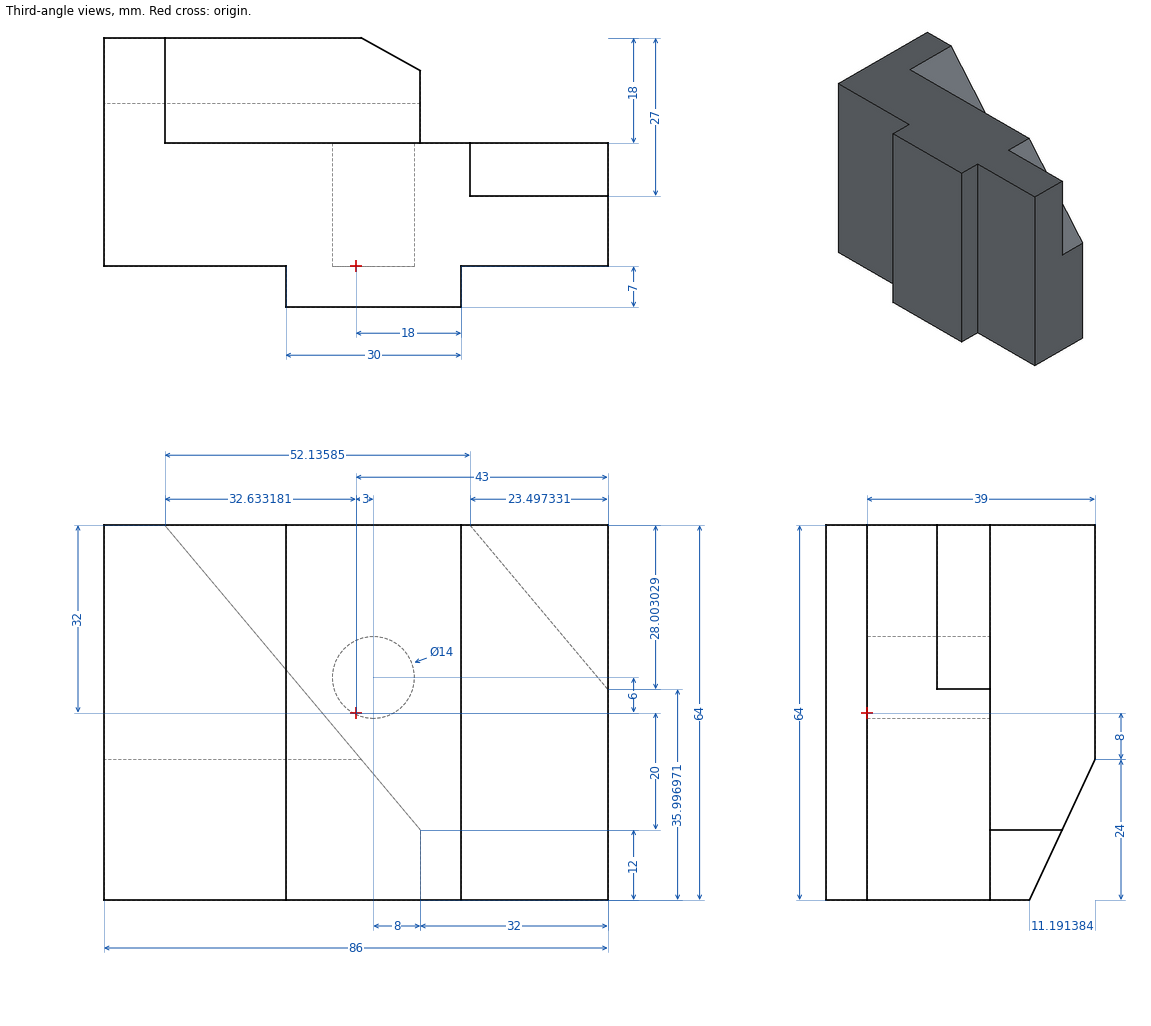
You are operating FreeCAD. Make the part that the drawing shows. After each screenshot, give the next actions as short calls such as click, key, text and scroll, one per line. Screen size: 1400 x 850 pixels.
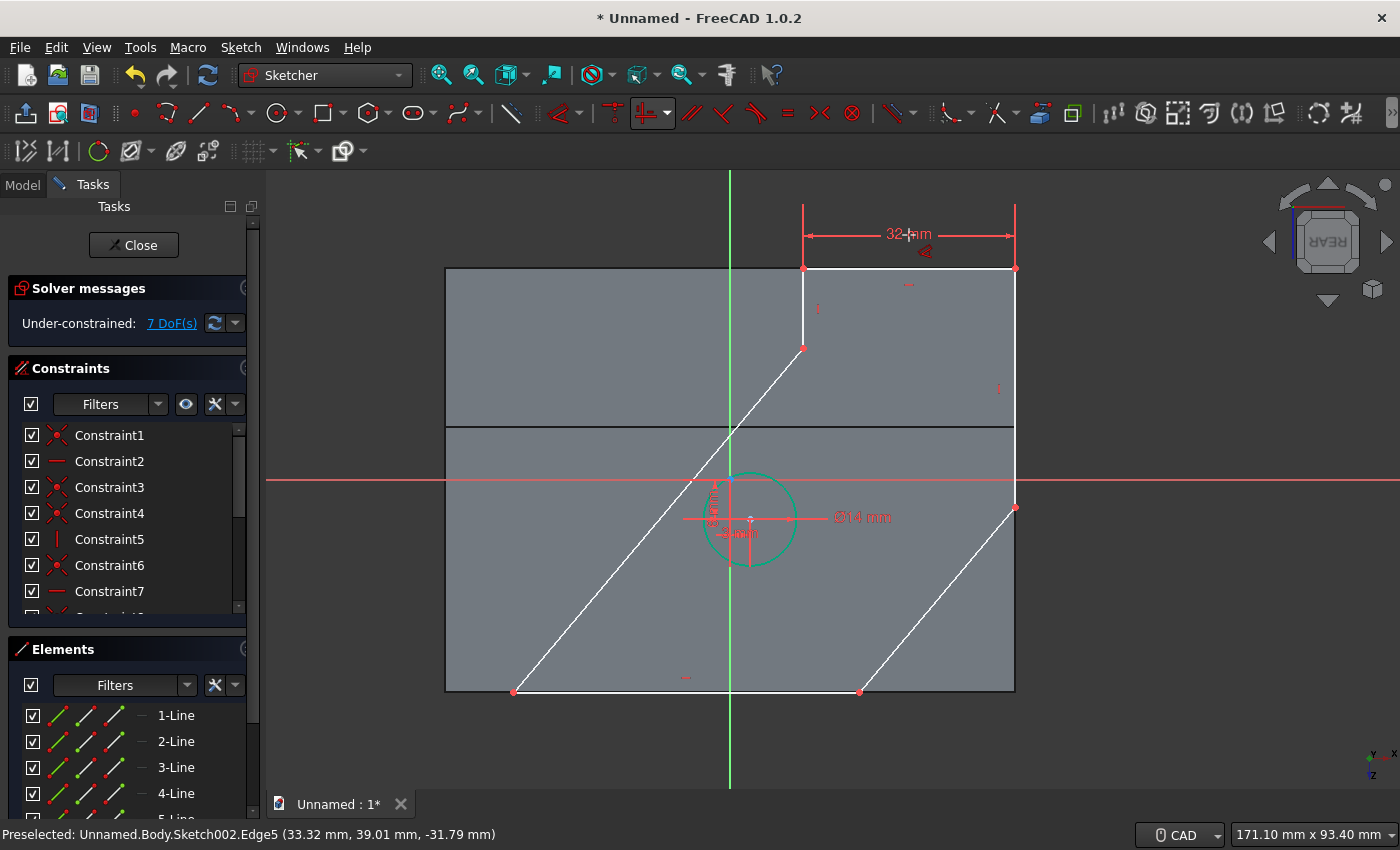
click(803, 293)
click(837, 309)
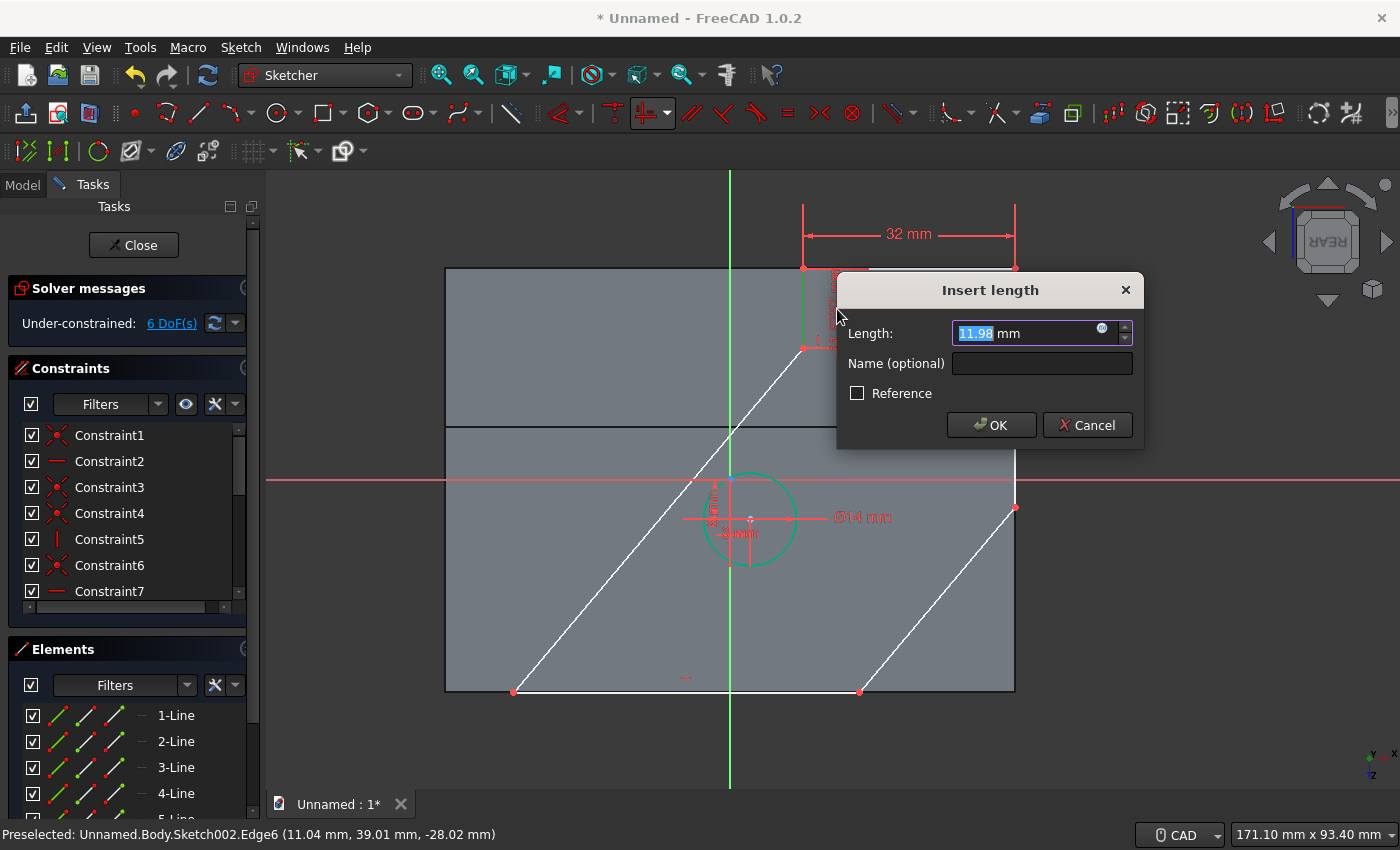
text(12)
key(Return)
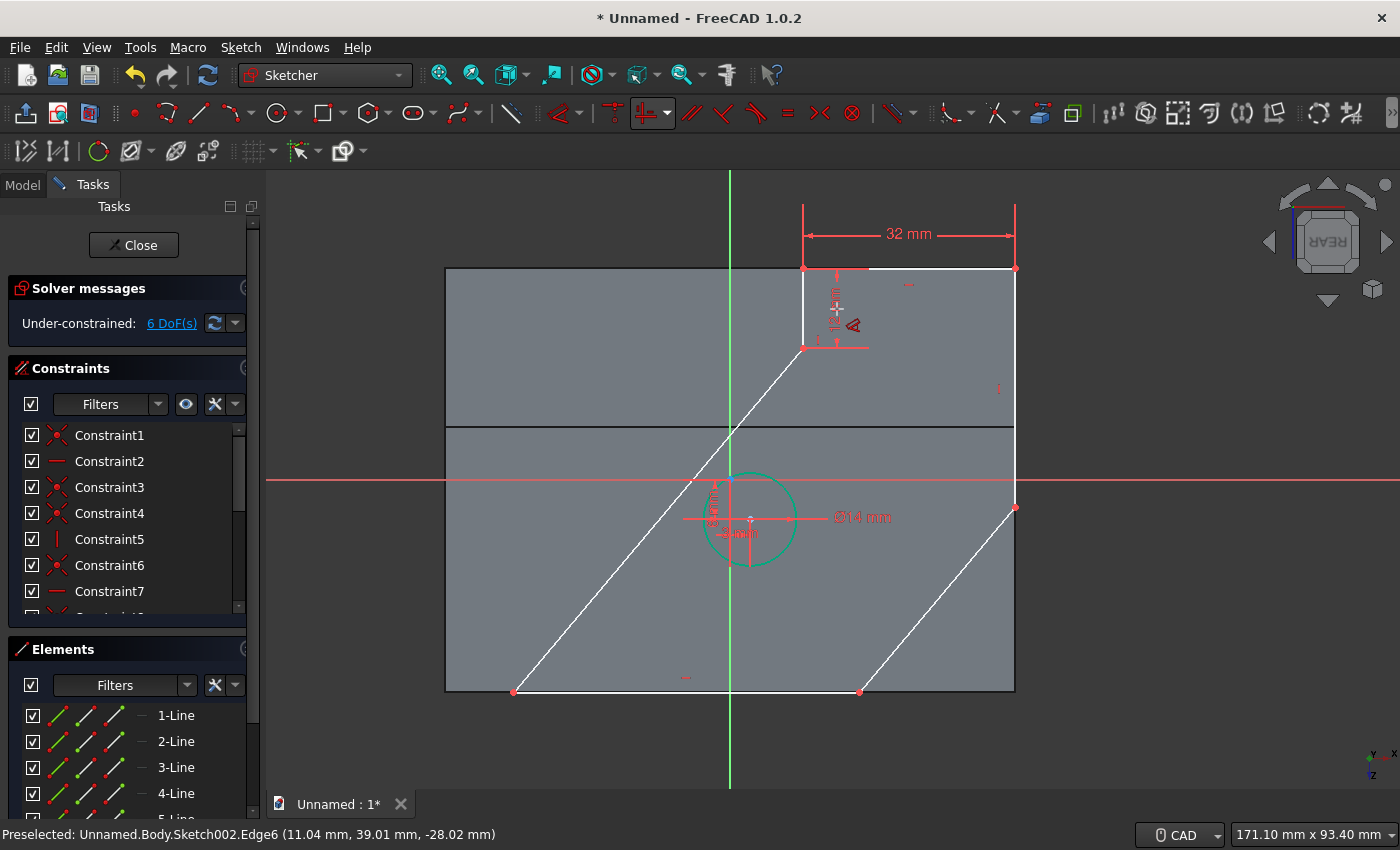
click(803, 348)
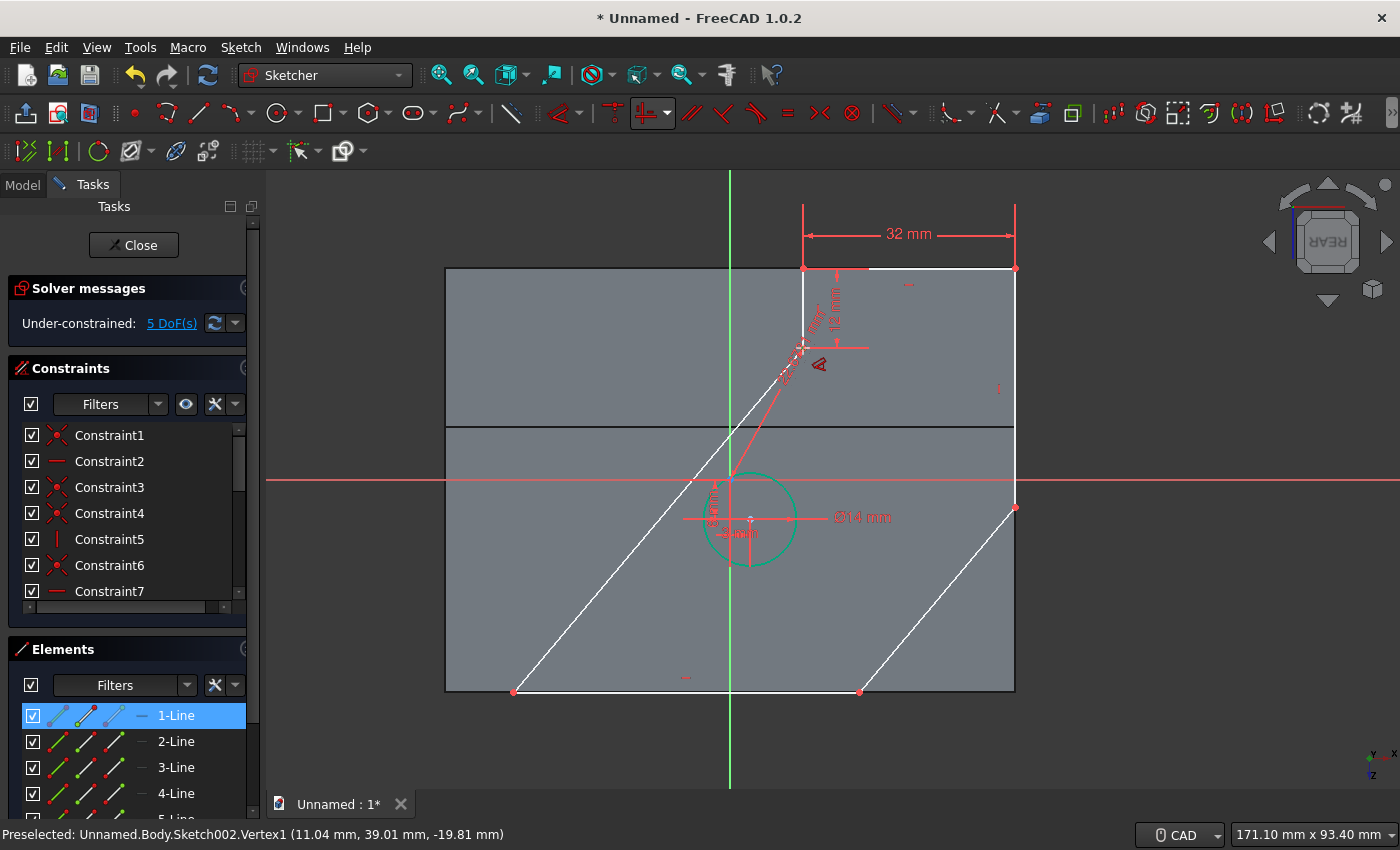
click(750, 519)
click(764, 314)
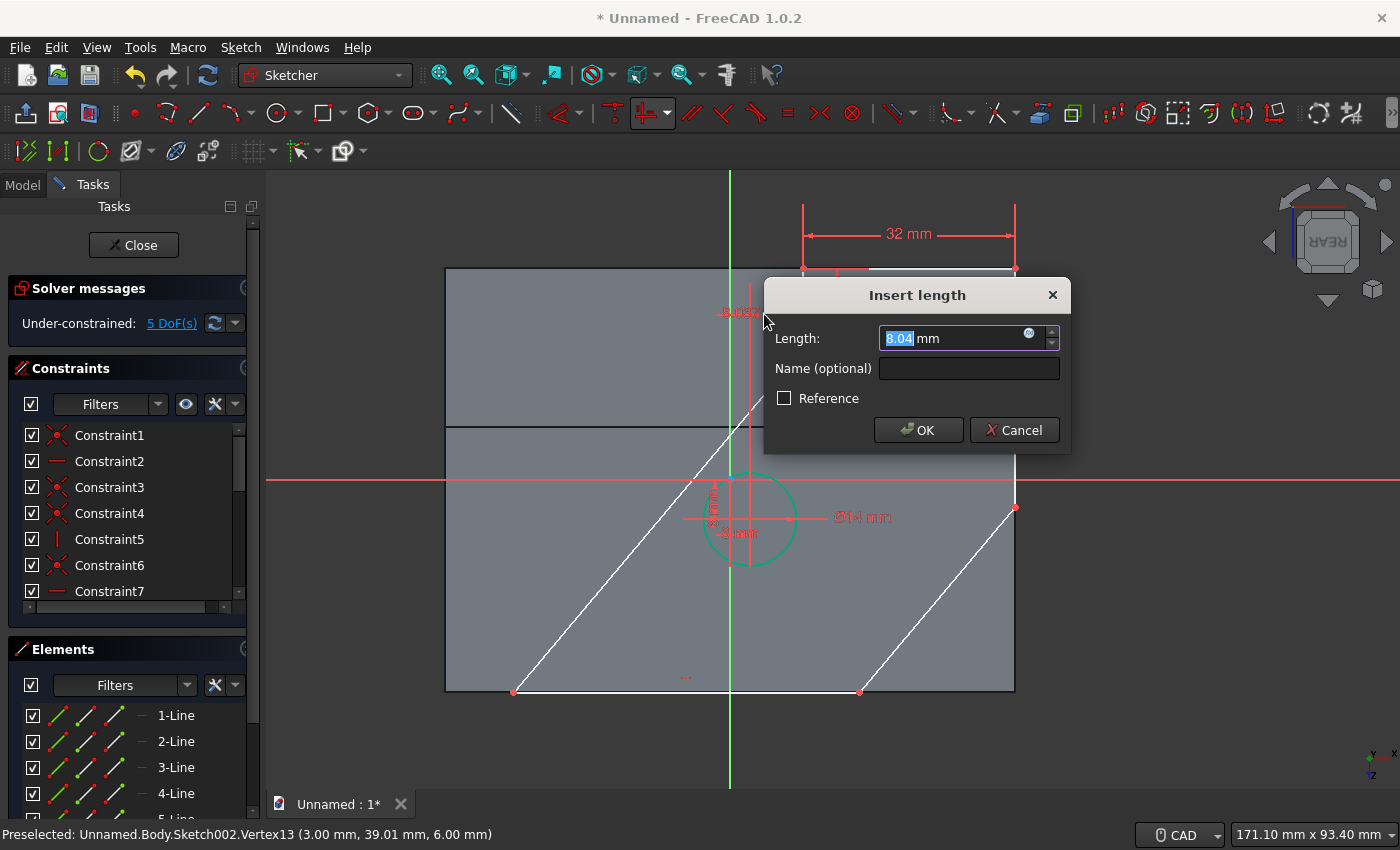
text(8)
key(Return)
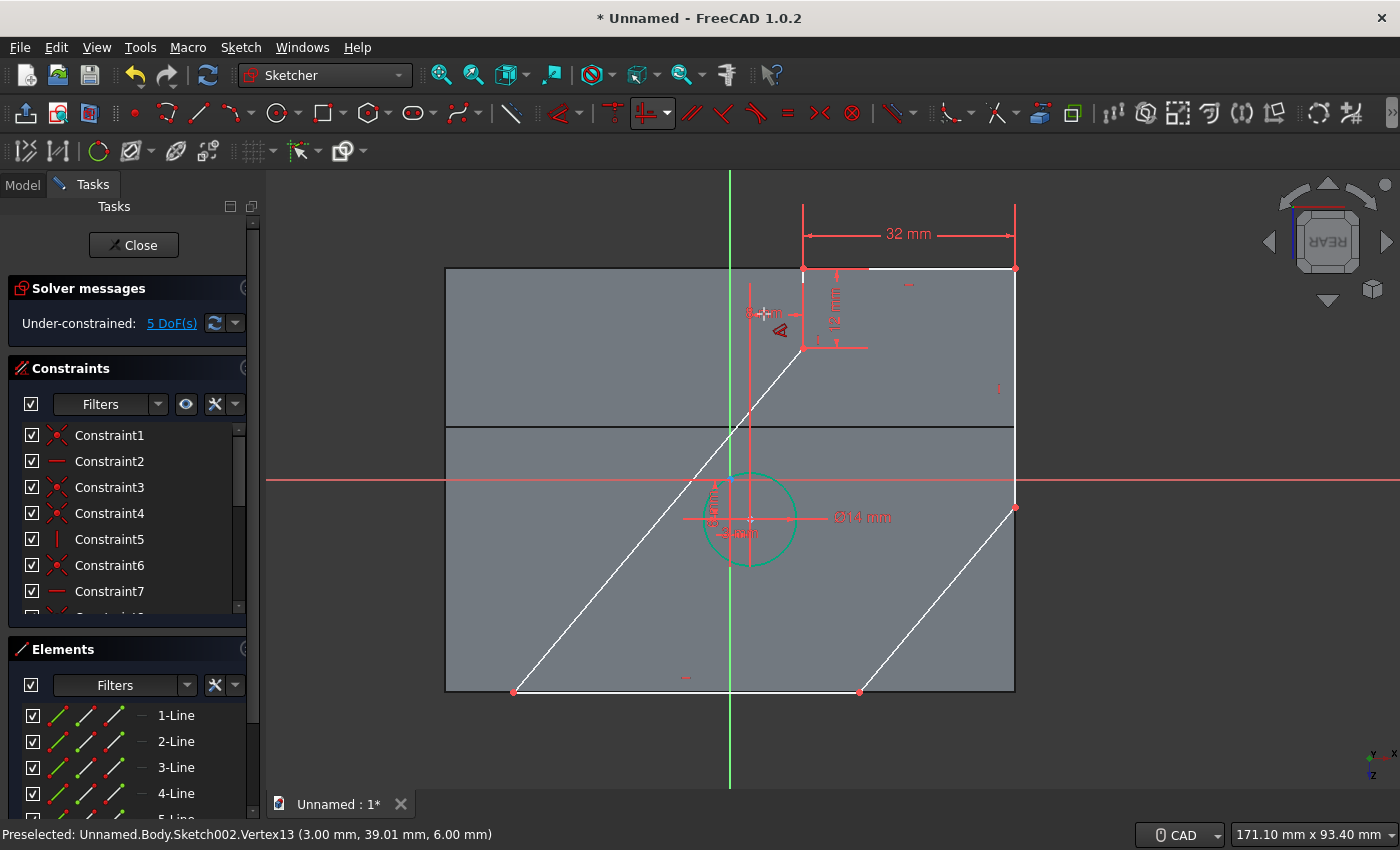
click(803, 348)
click(837, 414)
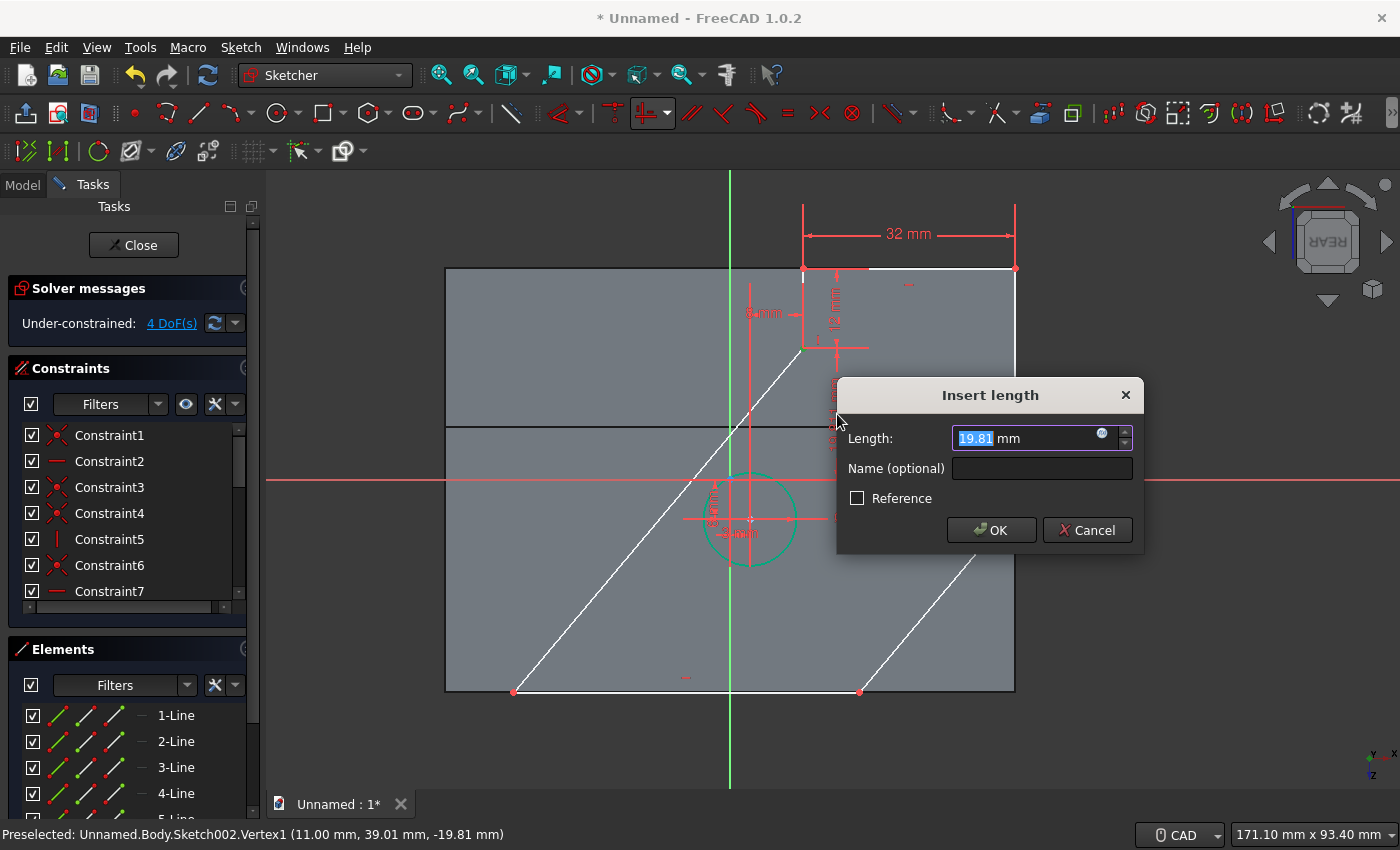
text(20)
key(Return)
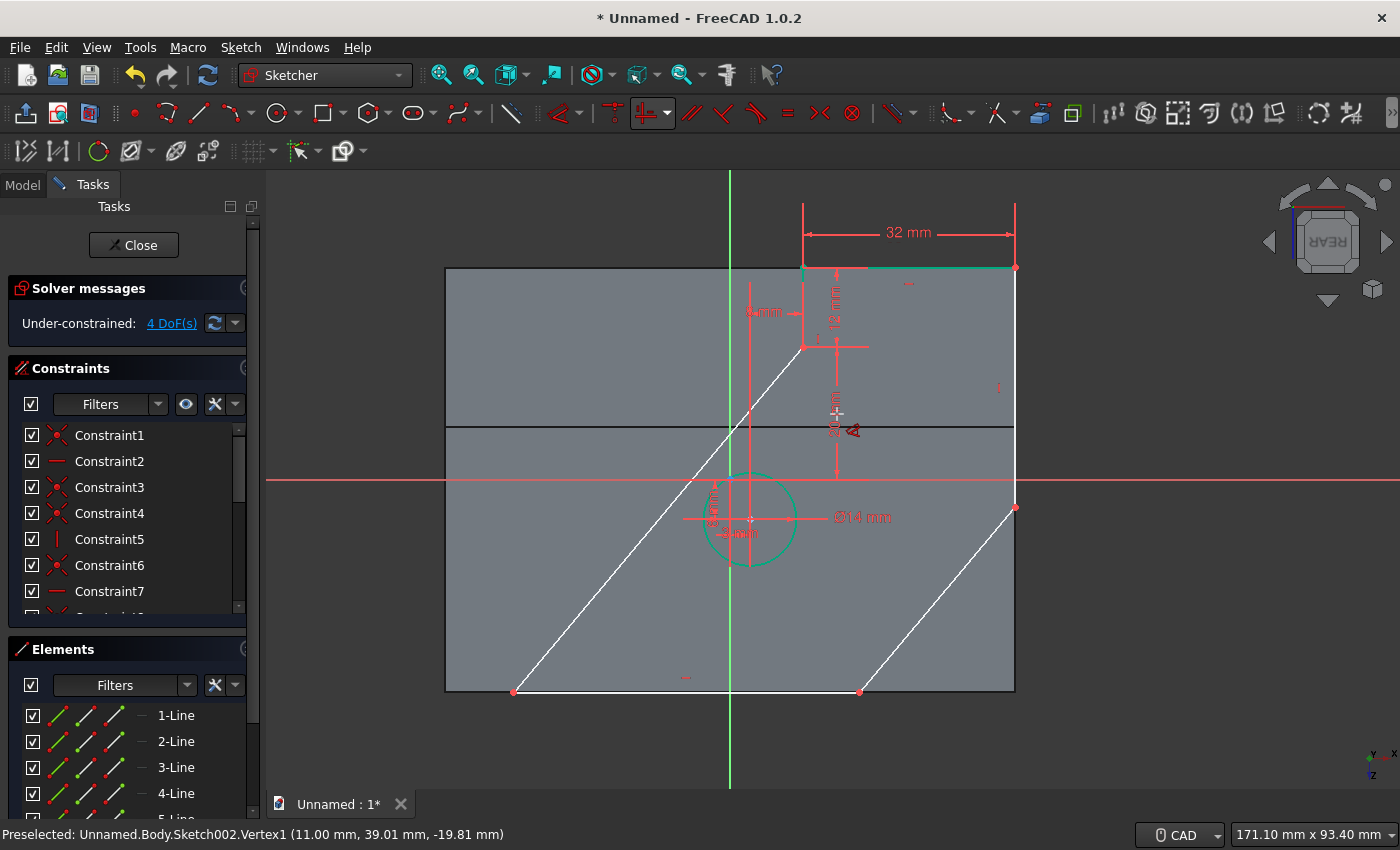
click(514, 693)
click(480, 586)